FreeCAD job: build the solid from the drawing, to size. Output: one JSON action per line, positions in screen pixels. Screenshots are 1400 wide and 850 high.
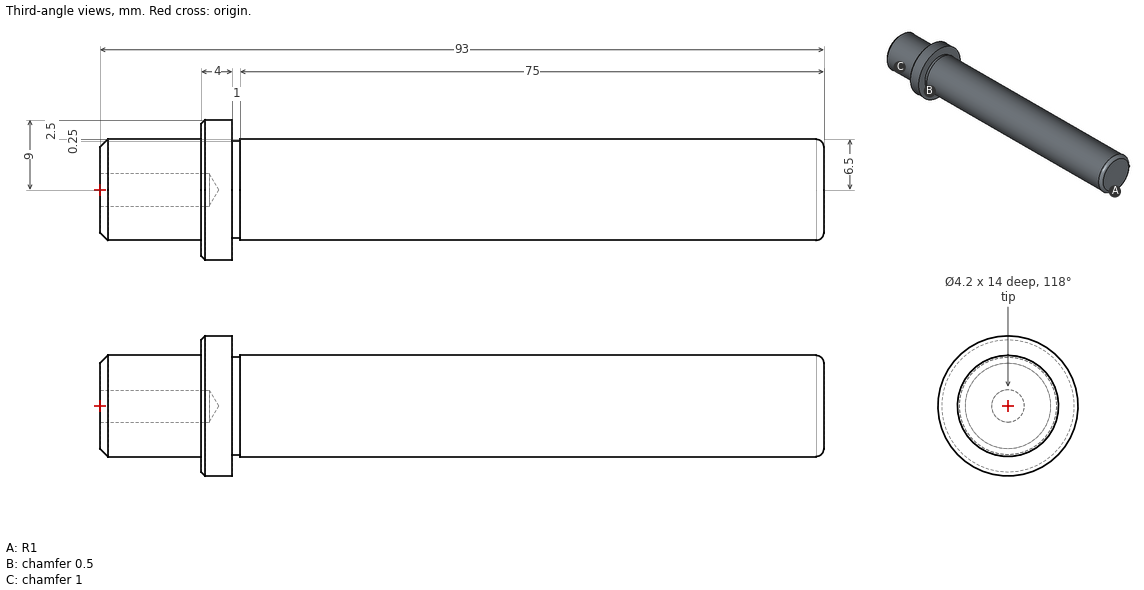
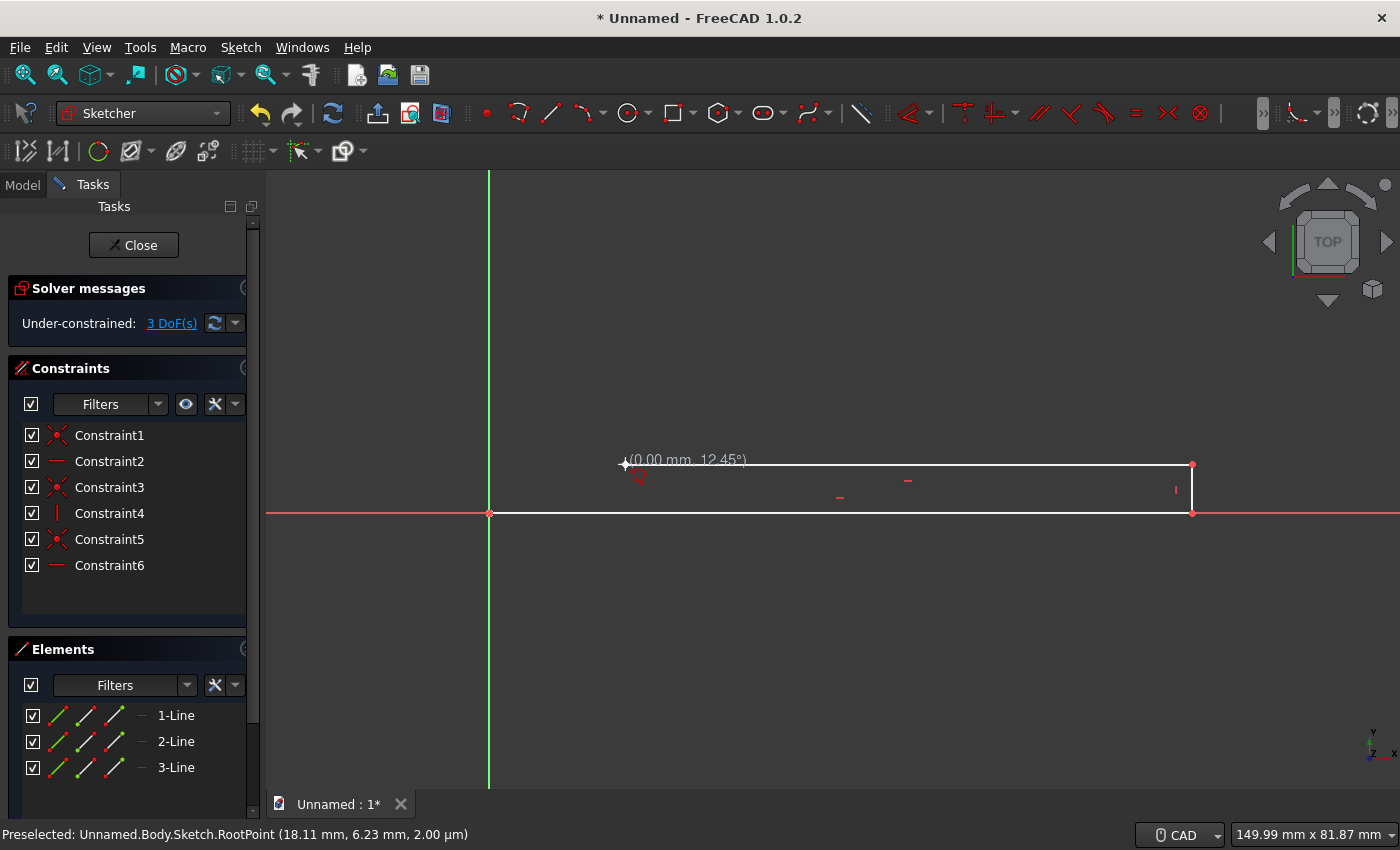
{"action": "scroll", "coordinate": [625, 466], "scroll_direction": "up", "scroll_amount": 11}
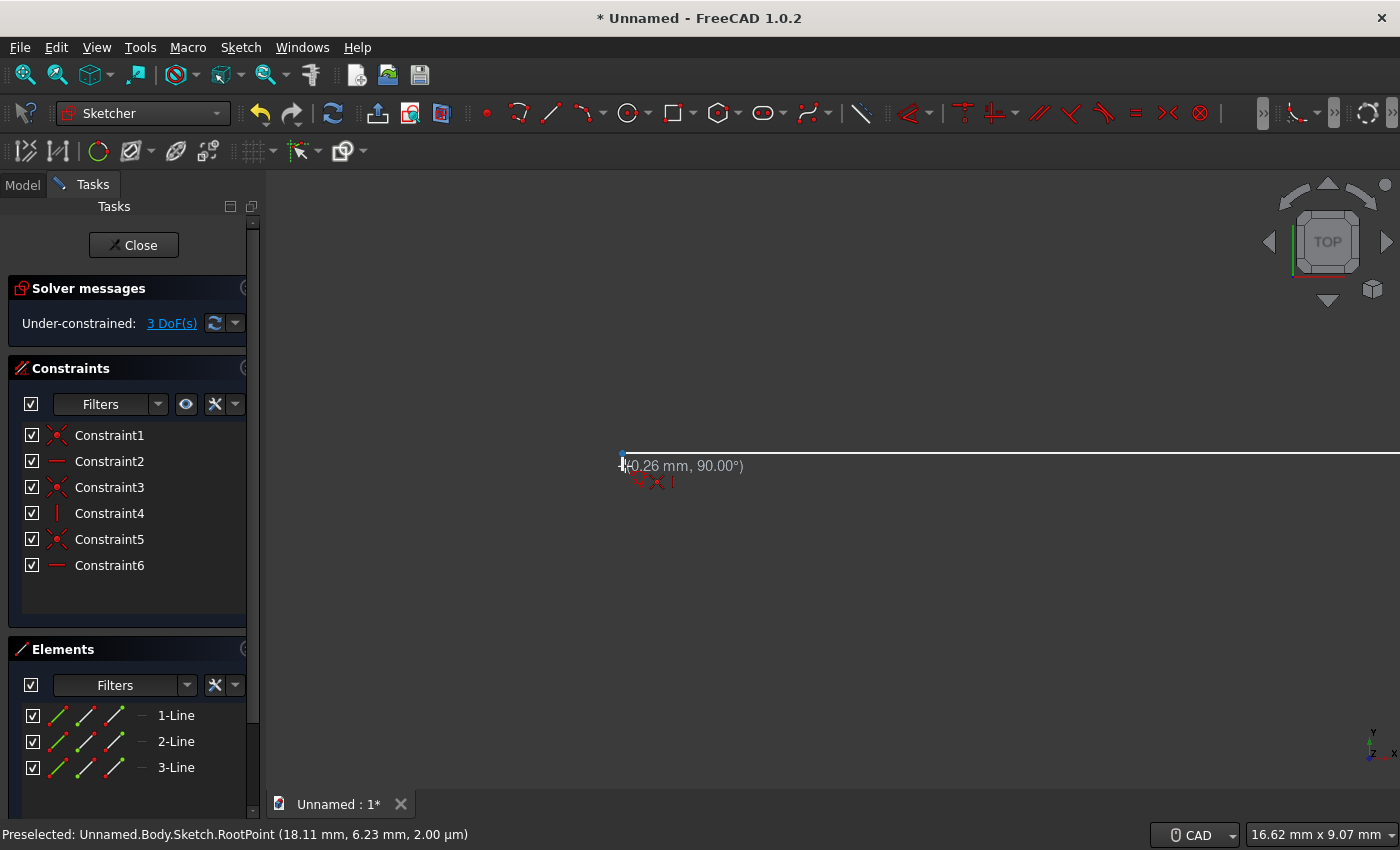
{"action": "left_click", "coordinate": [622, 461]}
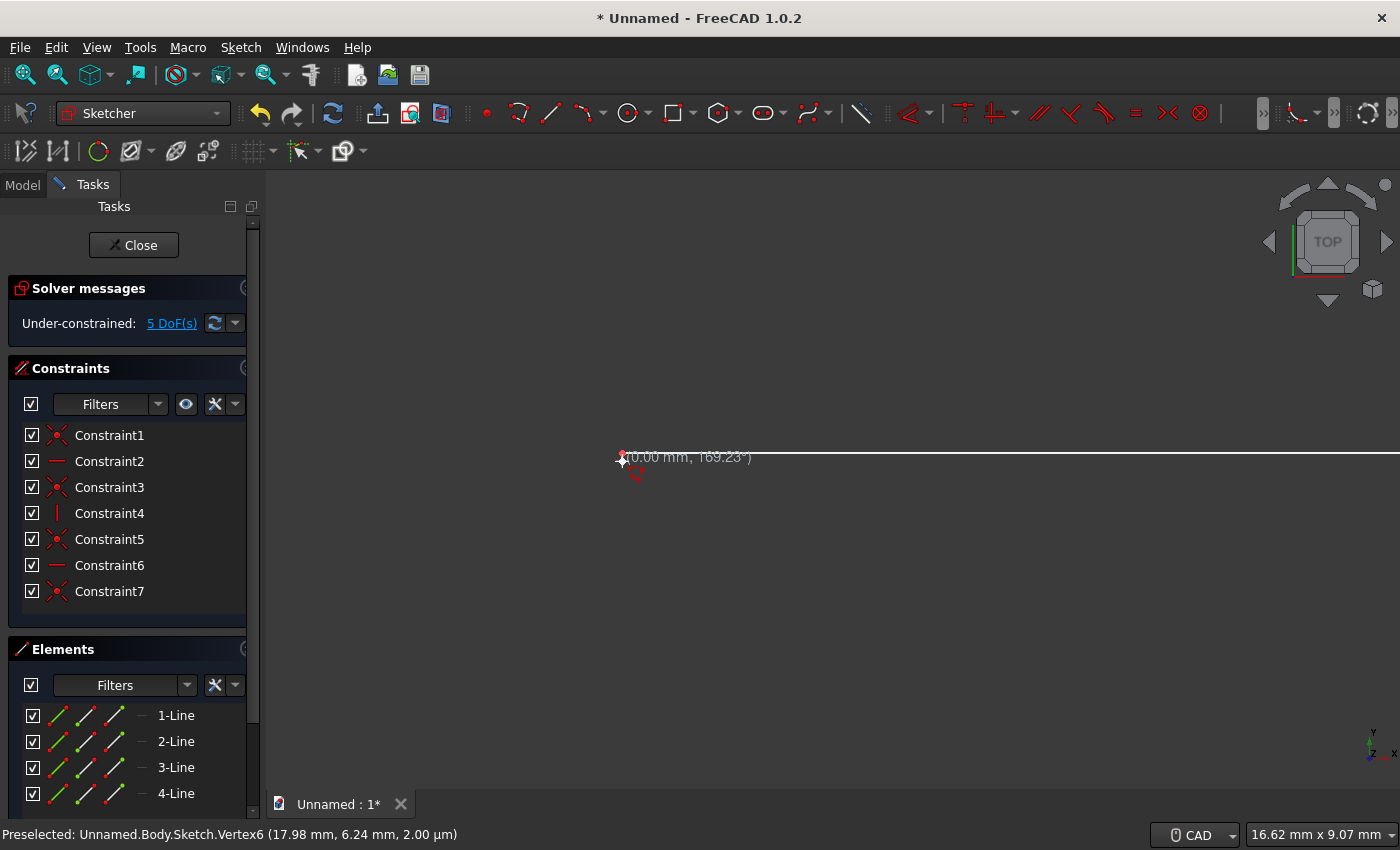
{"action": "scroll", "coordinate": [540, 467], "scroll_direction": "down", "scroll_amount": 11}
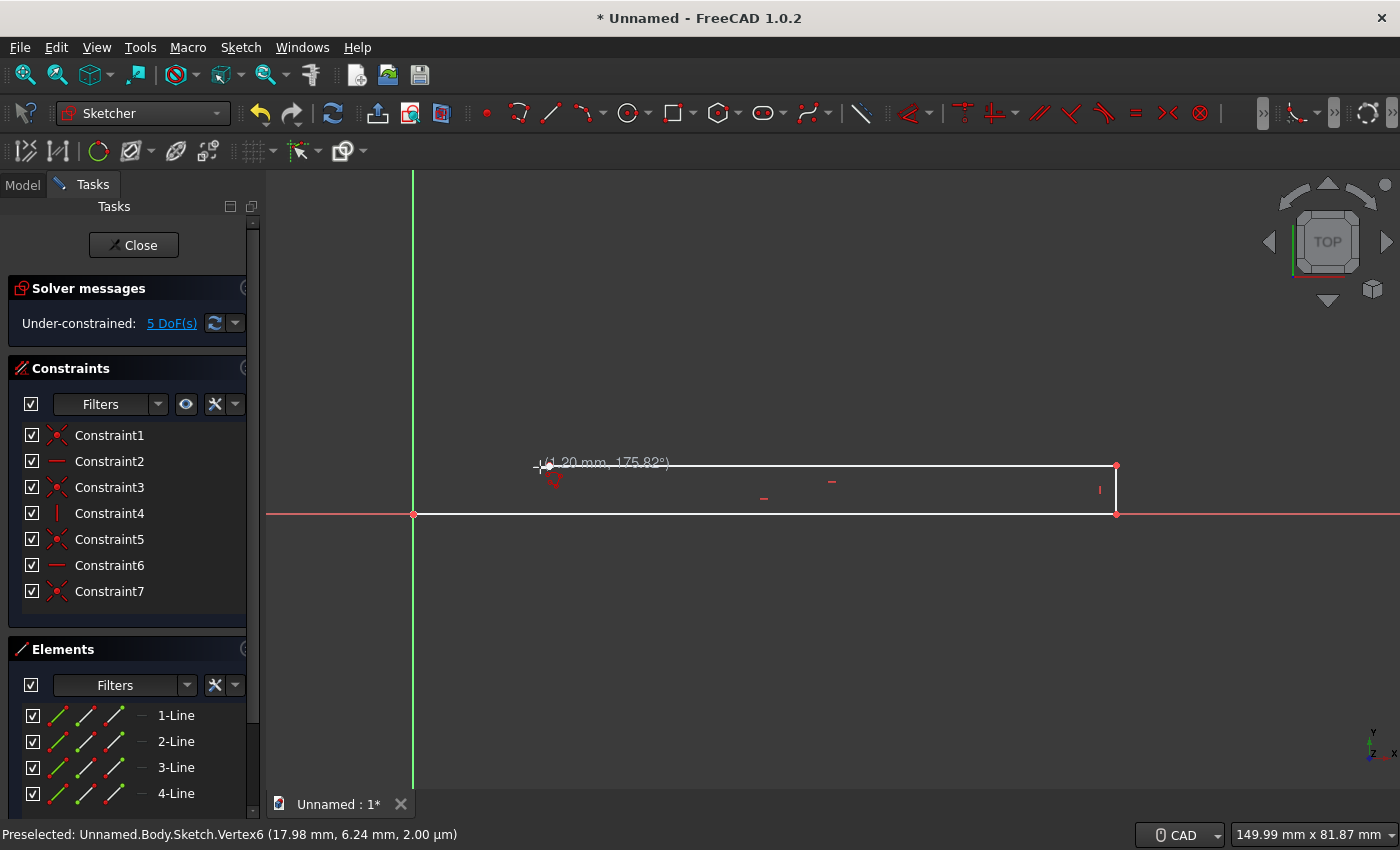
{"action": "scroll", "coordinate": [542, 467], "scroll_direction": "up", "scroll_amount": 4}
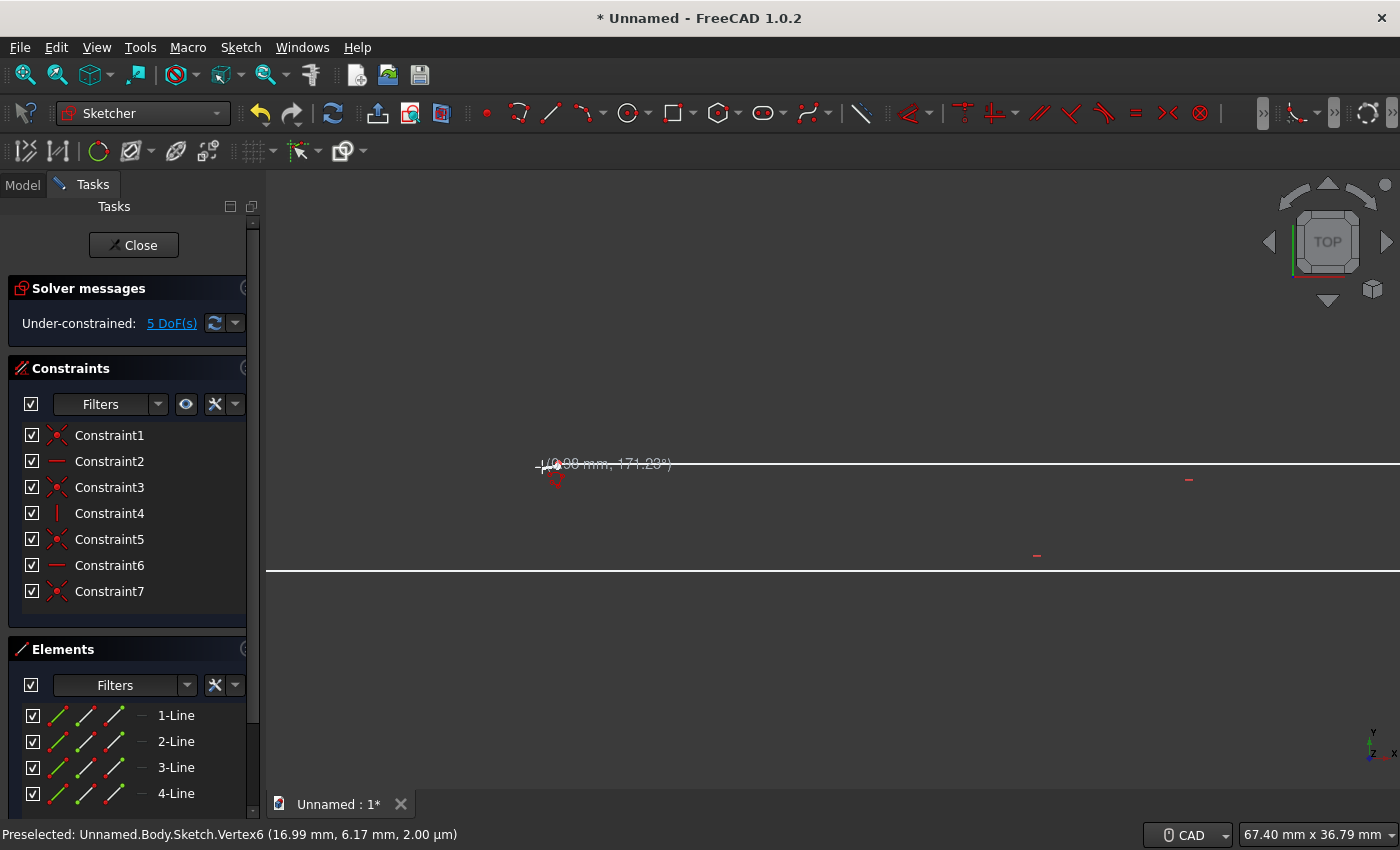
{"action": "left_click", "coordinate": [542, 466]}
{"action": "left_click", "coordinate": [542, 420]}
{"action": "left_click", "coordinate": [474, 420]}
{"action": "left_click", "coordinate": [474, 462]}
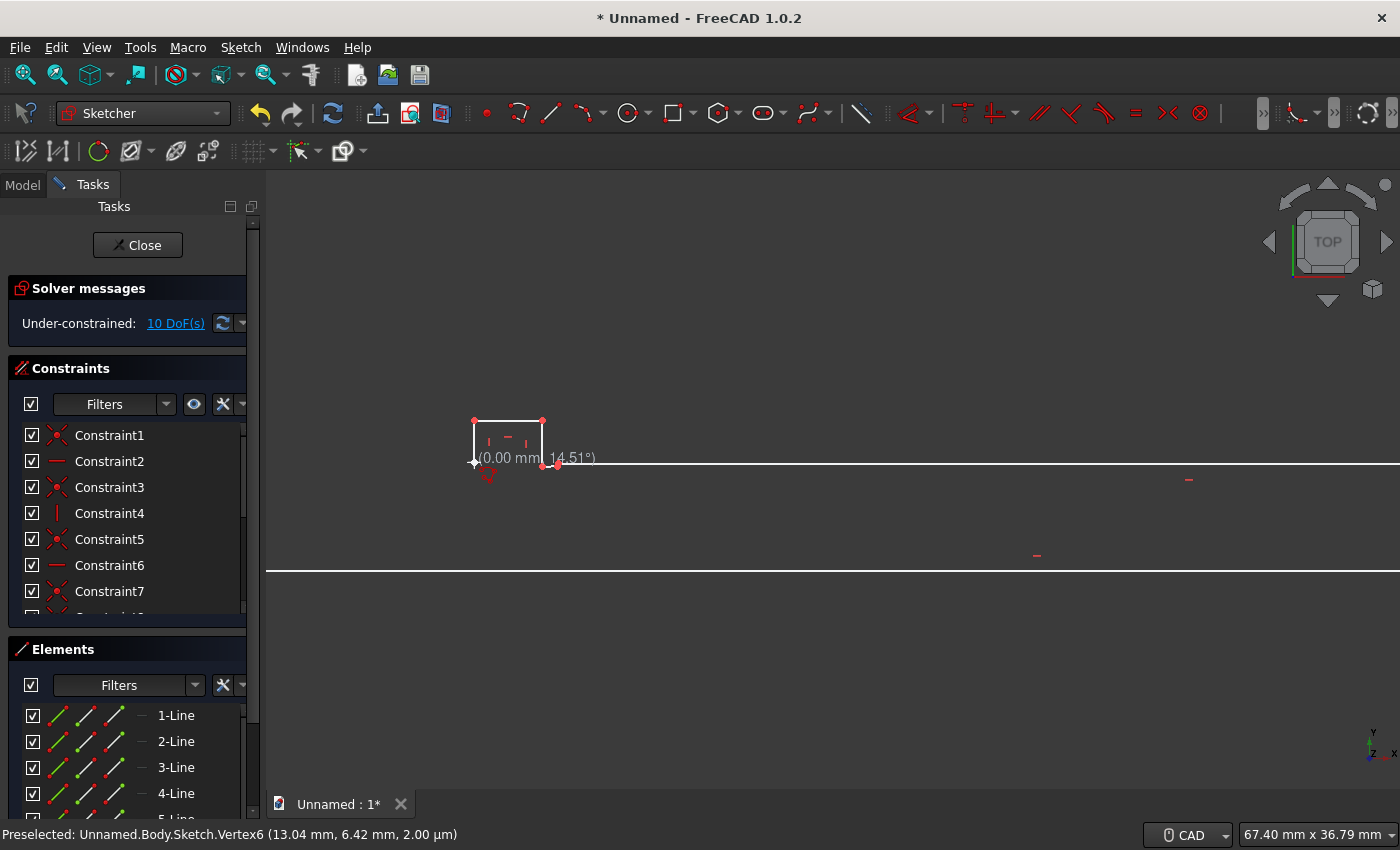
{"action": "scroll", "coordinate": [541, 467], "scroll_direction": "down", "scroll_amount": 4}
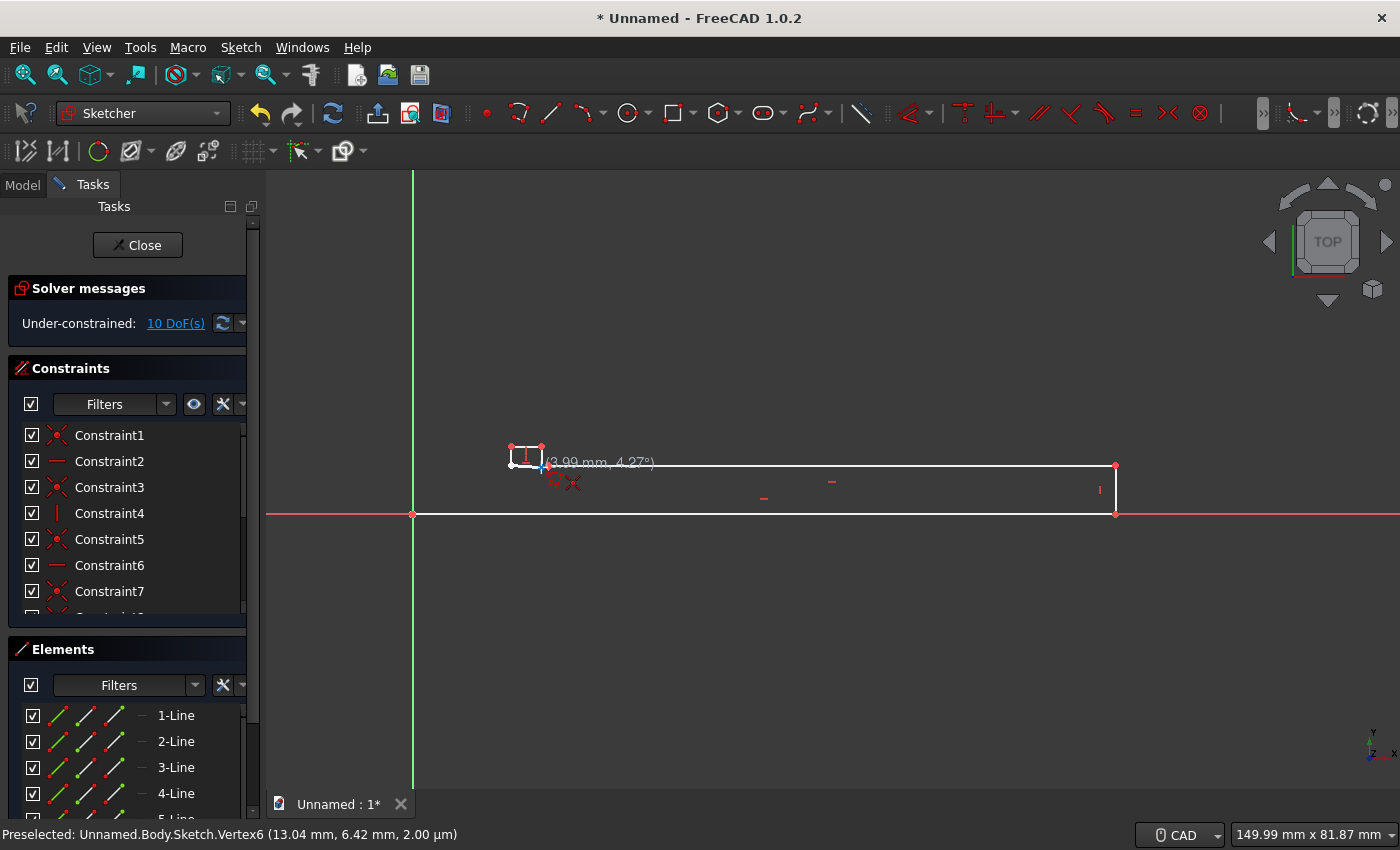
{"action": "left_click", "coordinate": [422, 465]}
{"action": "left_click", "coordinate": [413, 514]}
{"action": "key", "text": "Escape"}
{"action": "key", "text": "Escape"}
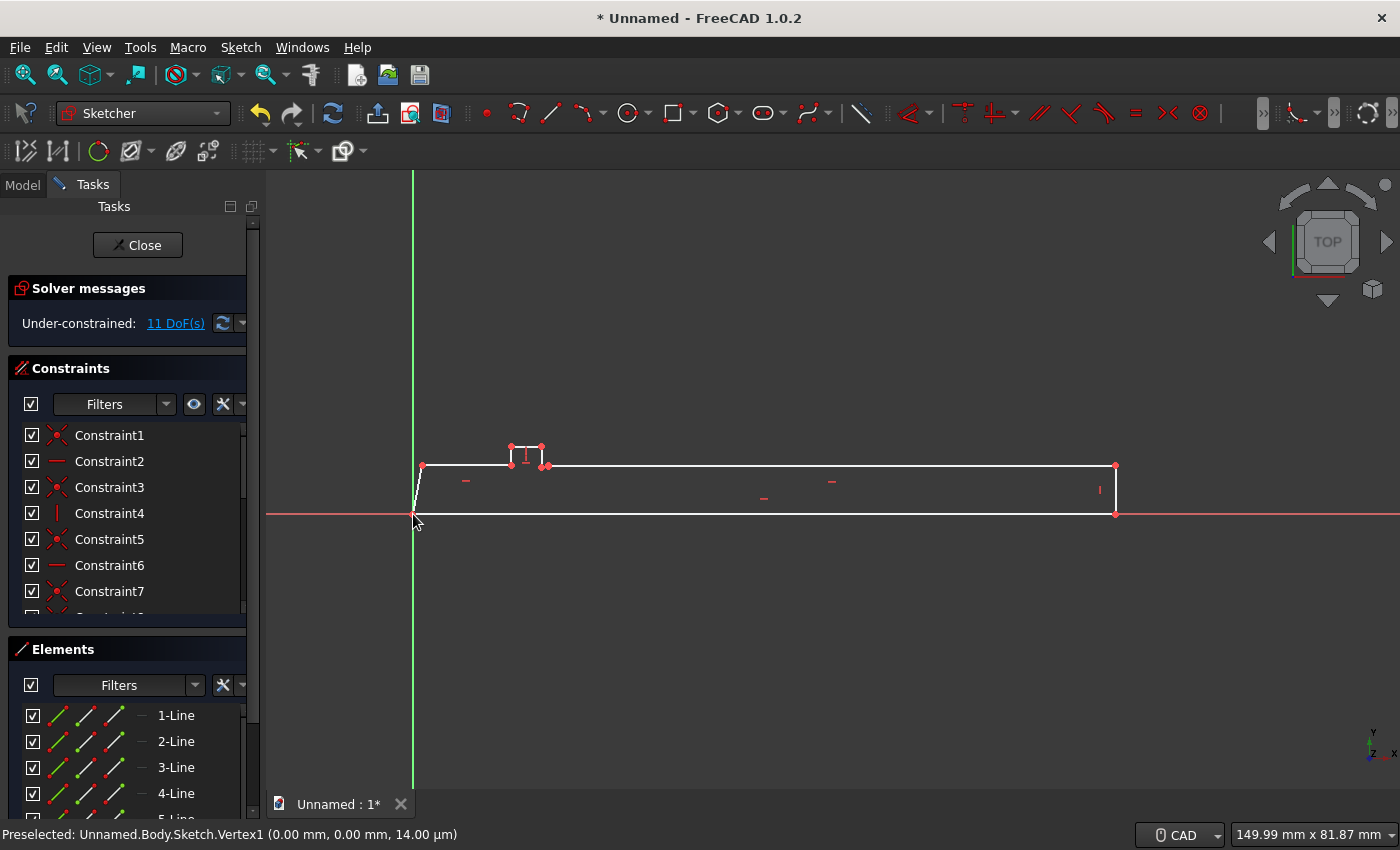
{"action": "scroll", "coordinate": [549, 466], "scroll_direction": "up", "scroll_amount": 14}